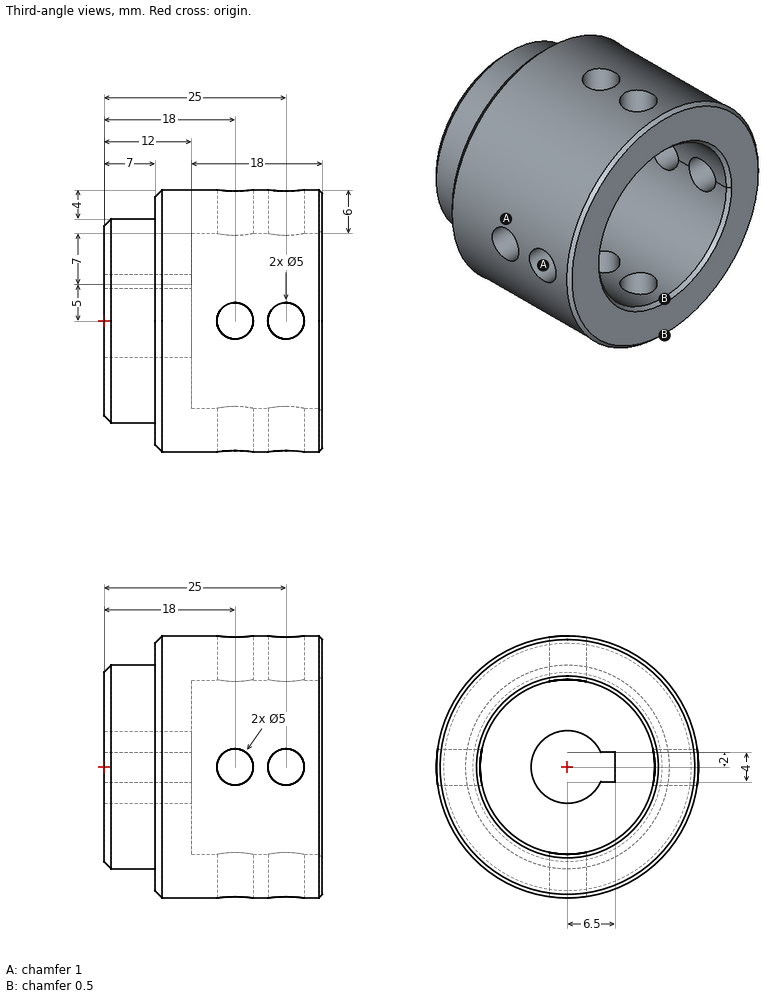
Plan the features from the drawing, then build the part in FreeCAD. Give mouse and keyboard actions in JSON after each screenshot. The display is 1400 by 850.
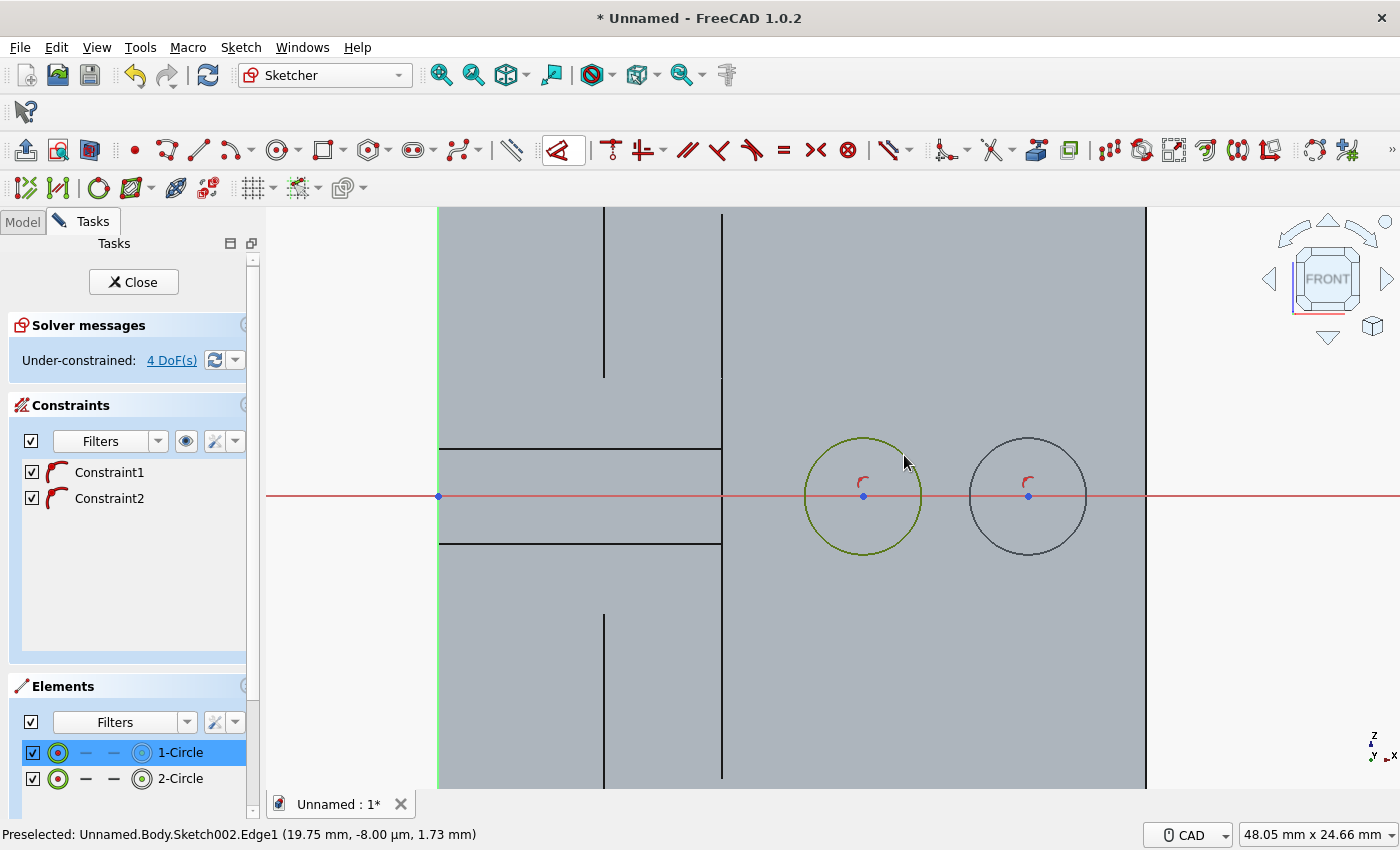
{"action": "left_click", "coordinate": [1069, 455]}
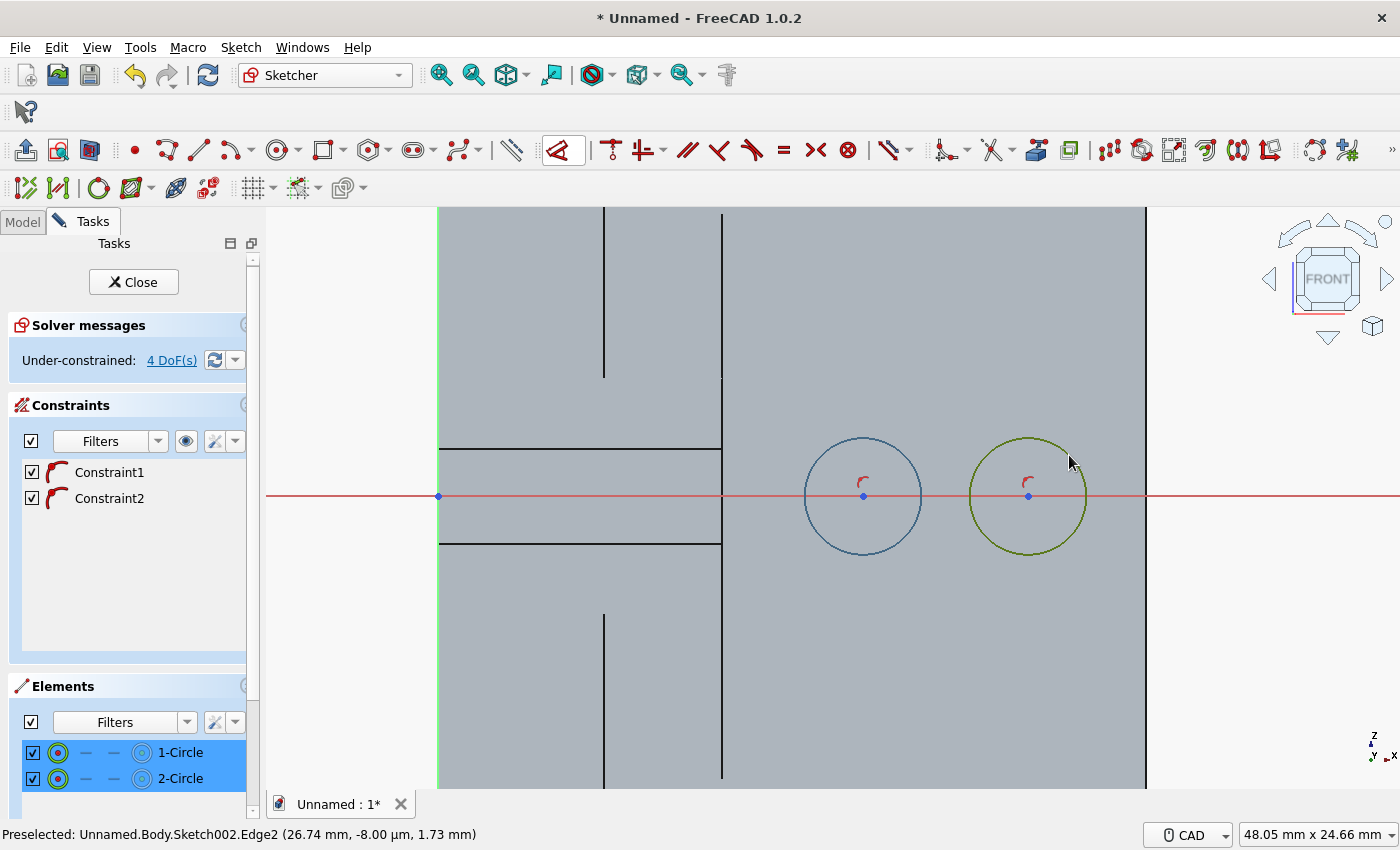
{"action": "left_click", "coordinate": [784, 150]}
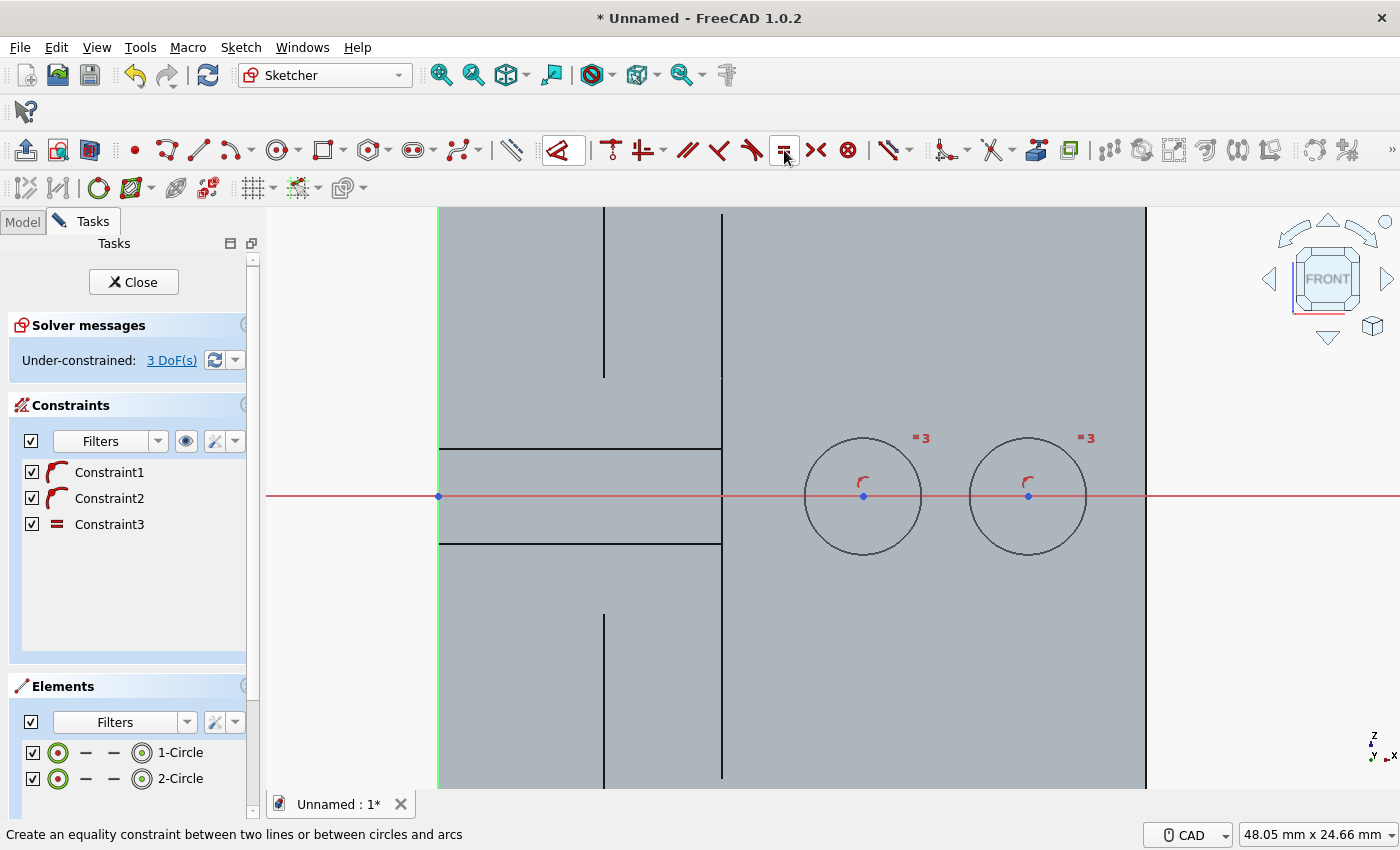
{"action": "left_click", "coordinate": [904, 455]}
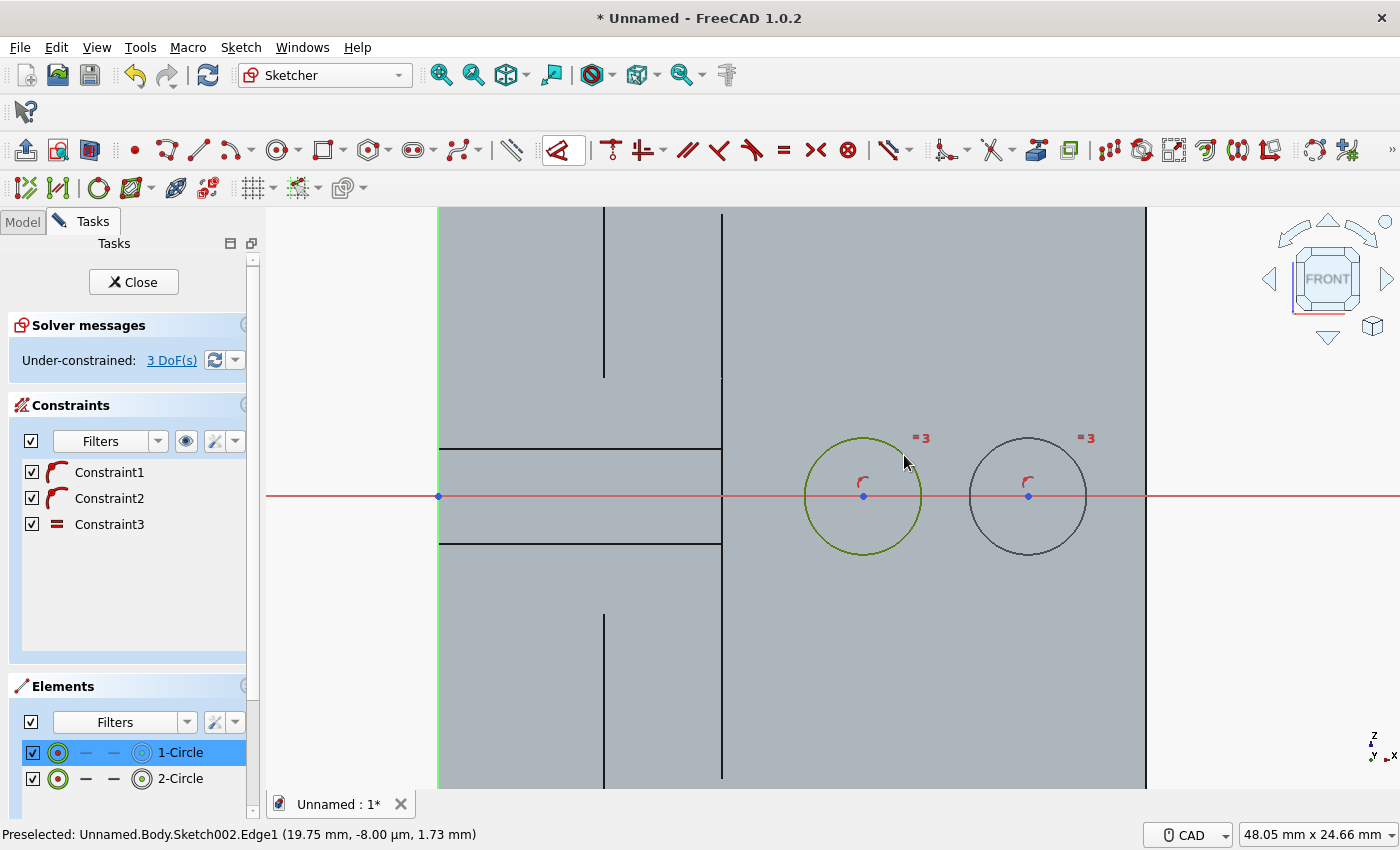
{"action": "left_click", "coordinate": [580, 150]}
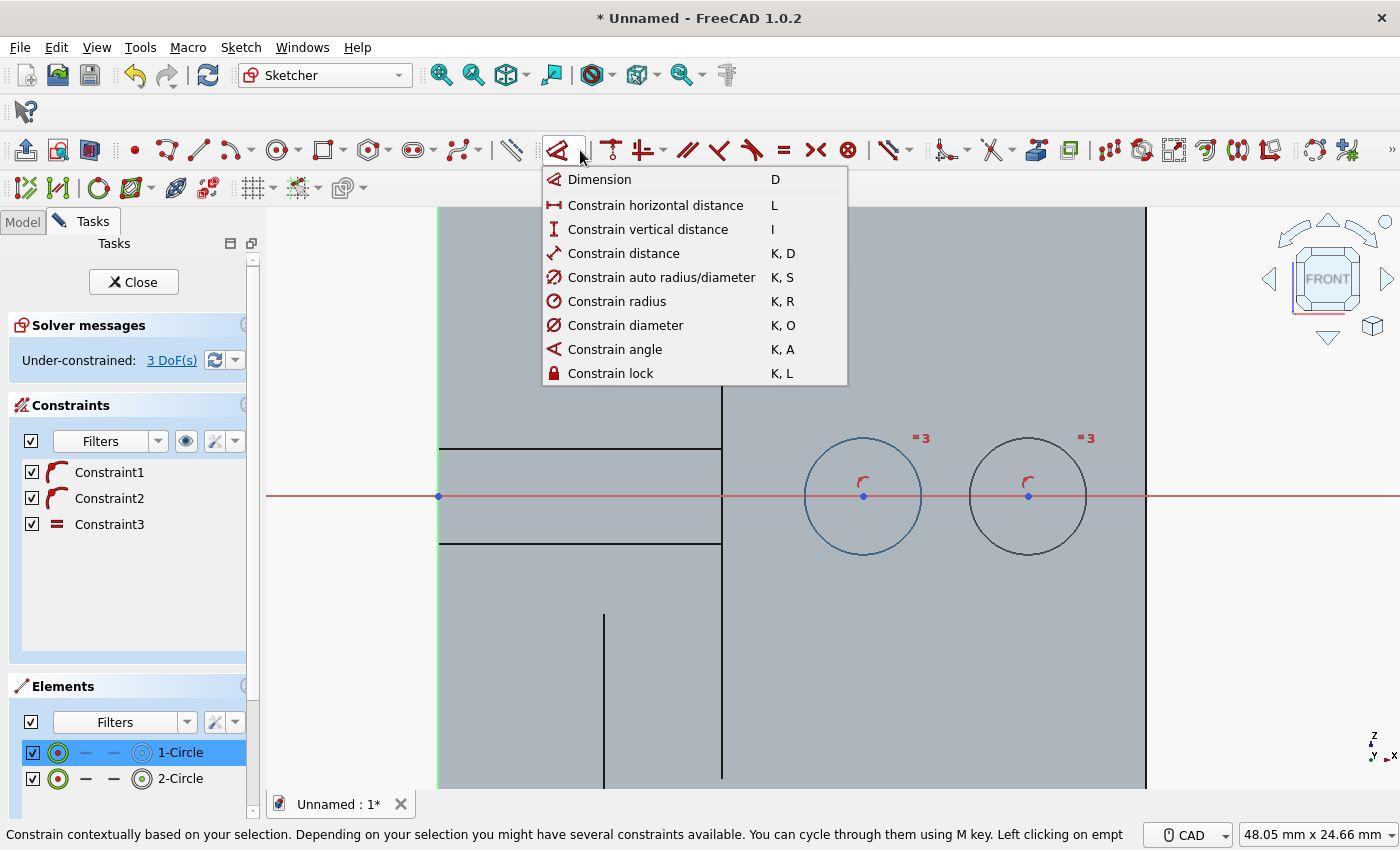
{"action": "left_click", "coordinate": [695, 325]}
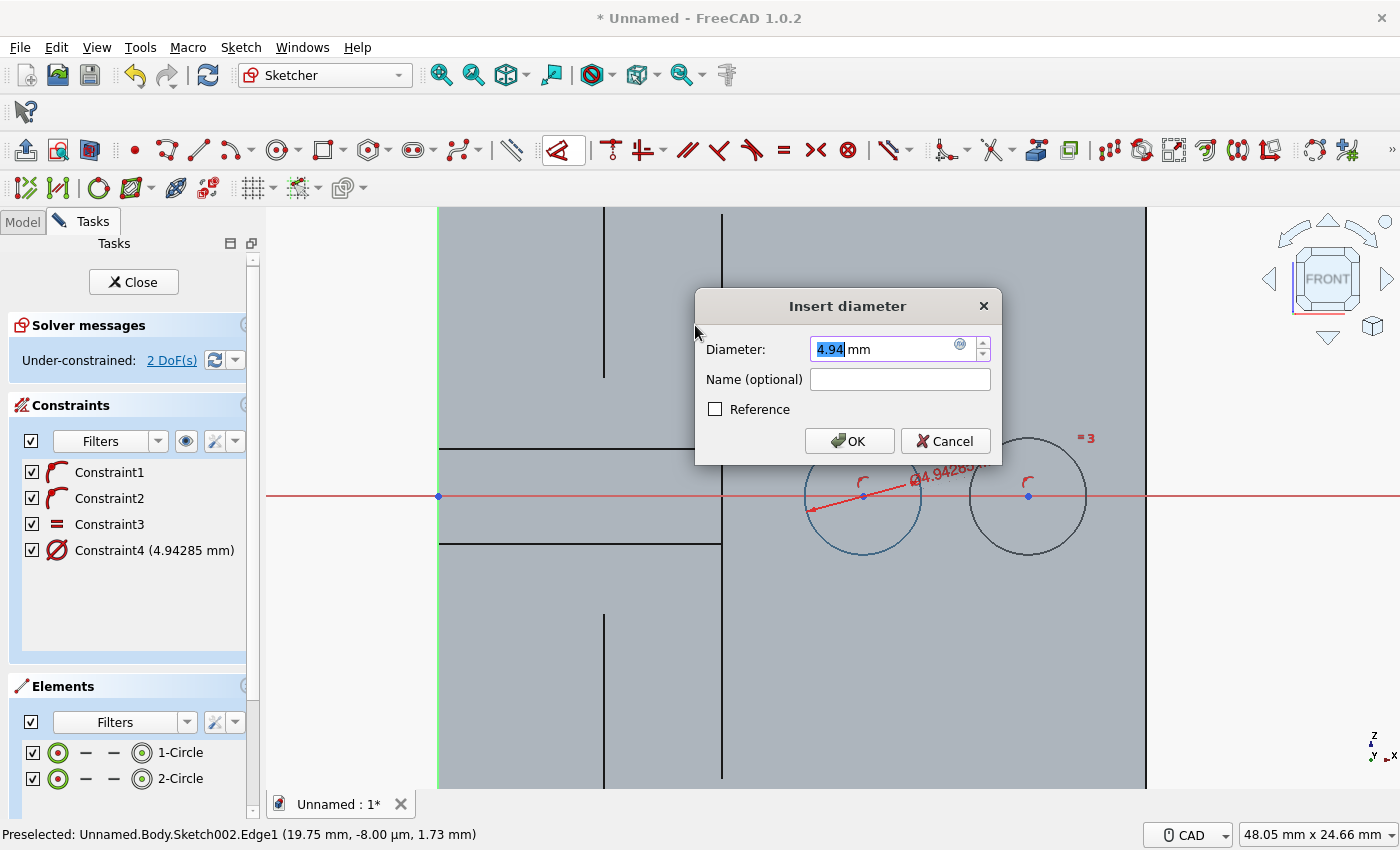
{"action": "type", "text": "5"}
{"action": "key", "text": "Return"}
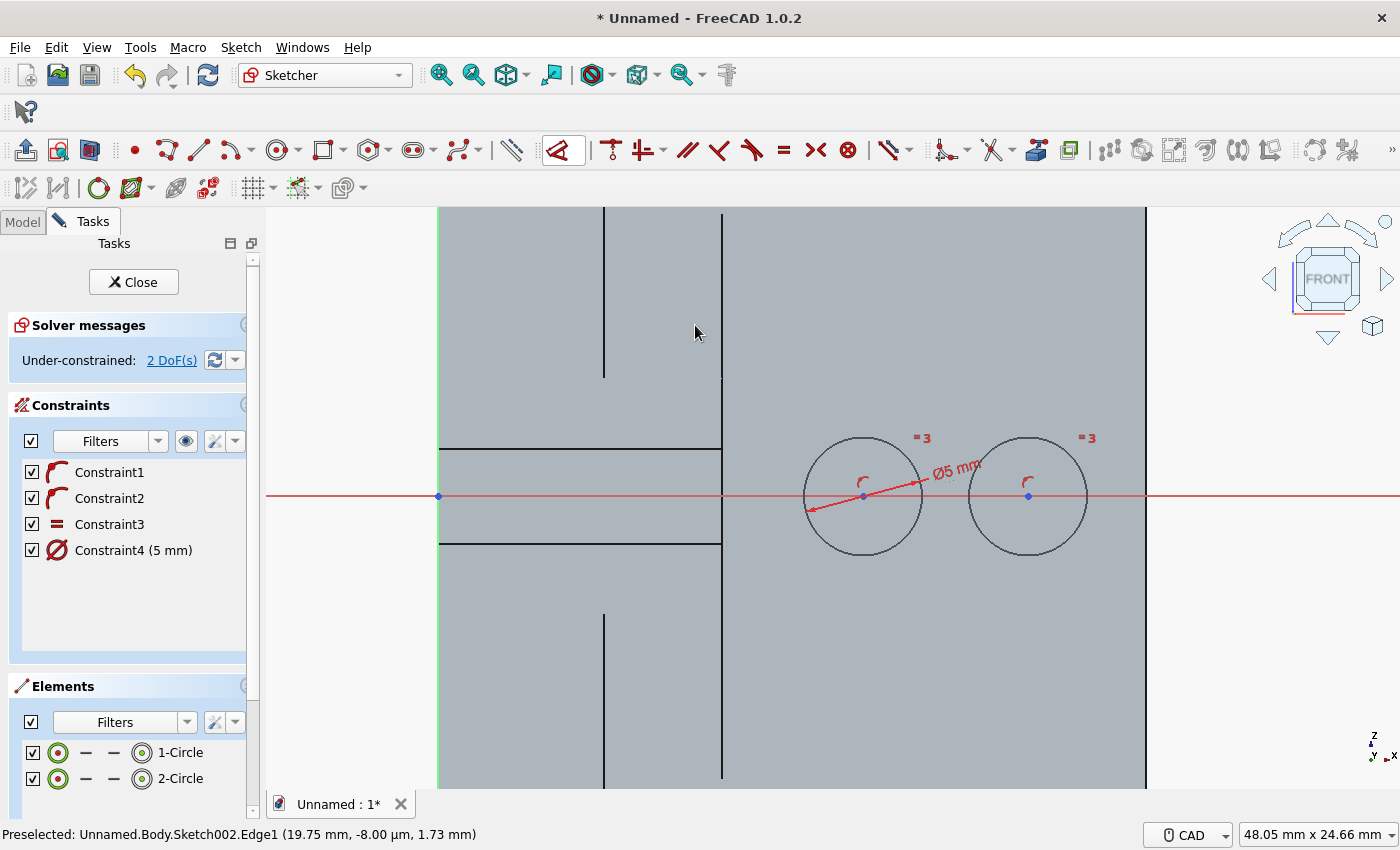
{"action": "left_click", "coordinate": [863, 496]}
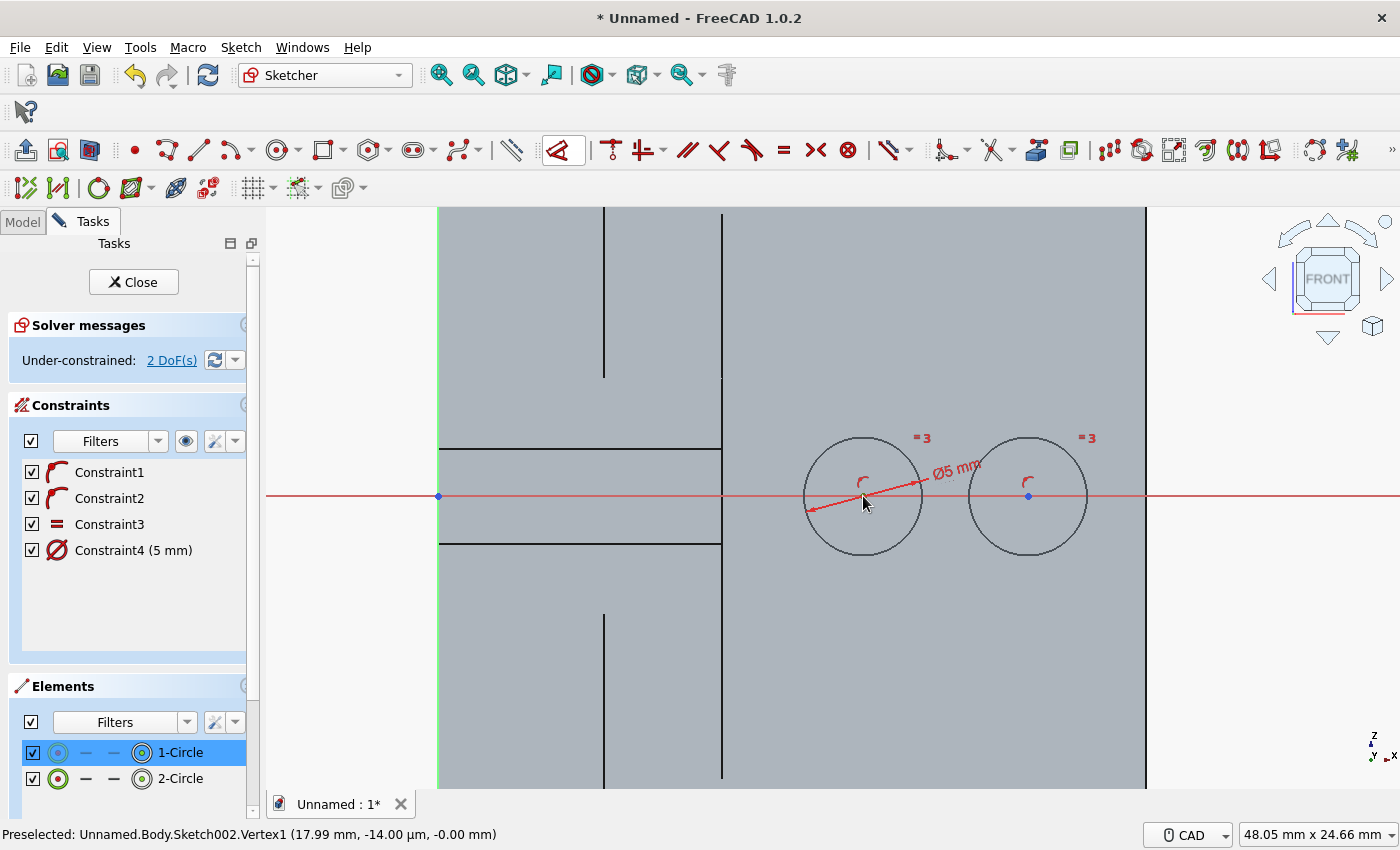
{"action": "key", "text": "l"}